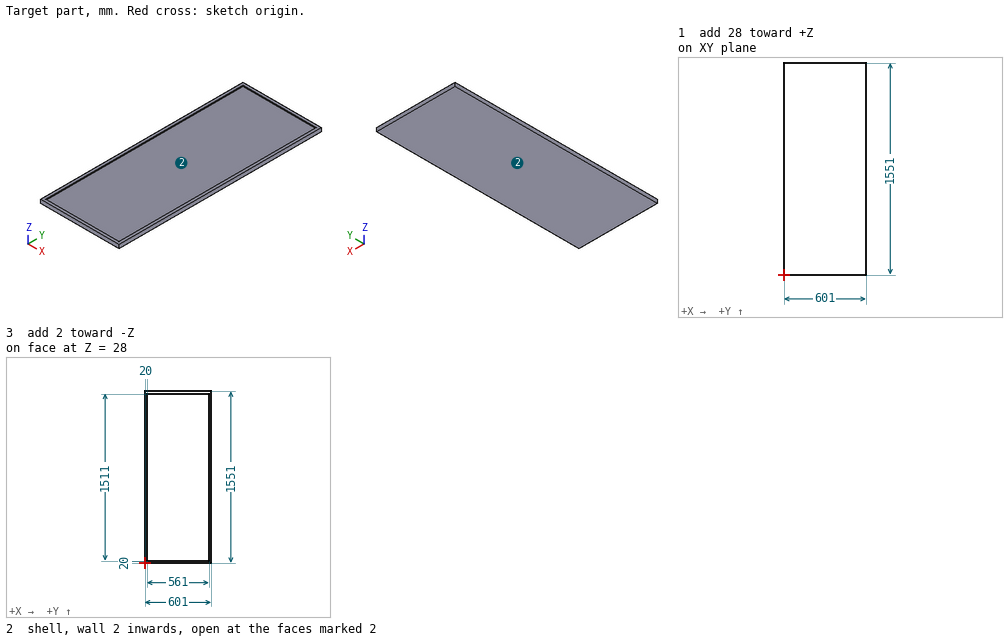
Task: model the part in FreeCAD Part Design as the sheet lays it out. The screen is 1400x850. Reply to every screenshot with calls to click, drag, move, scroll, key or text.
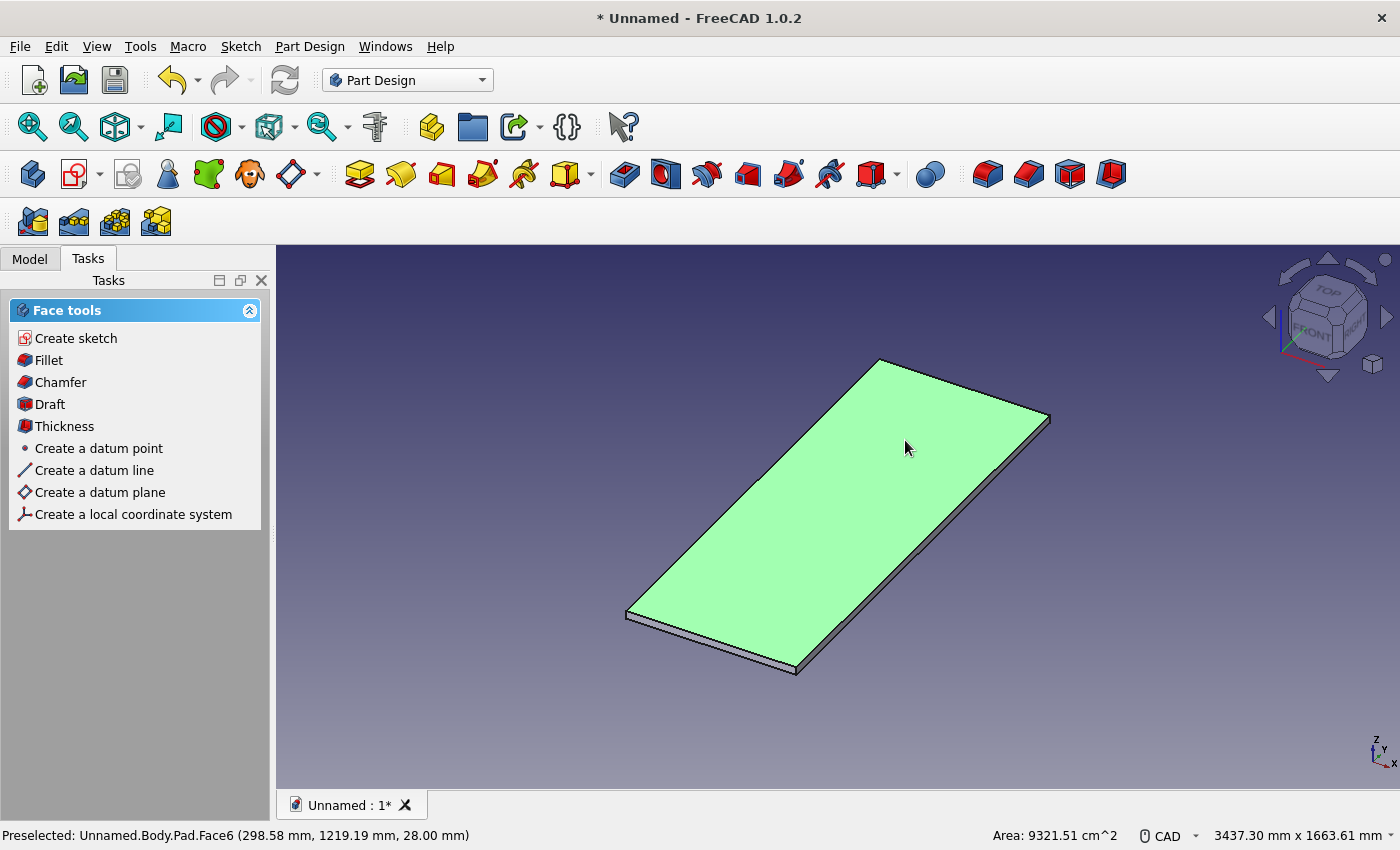
click(1111, 174)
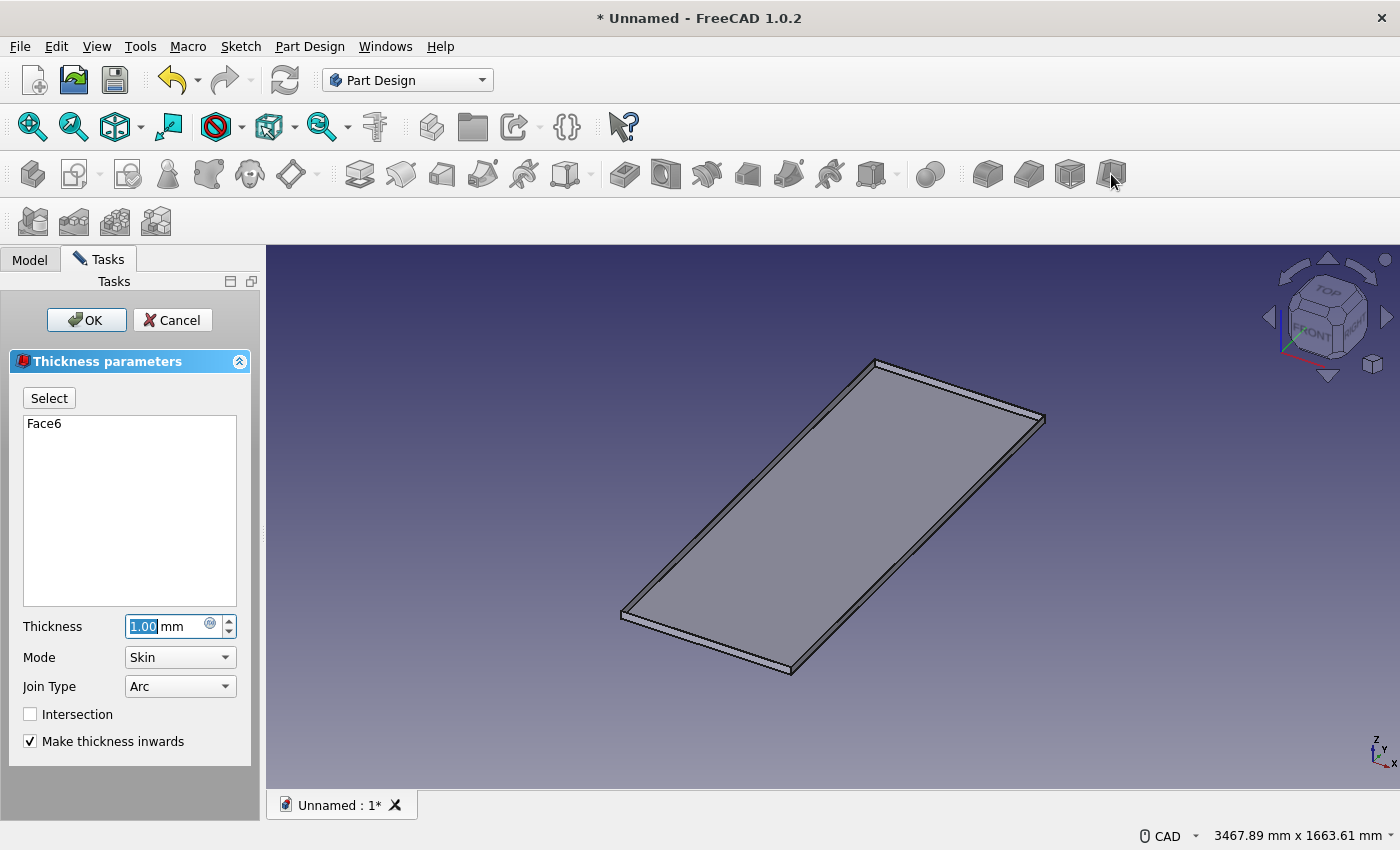
text(2)
key(Tab)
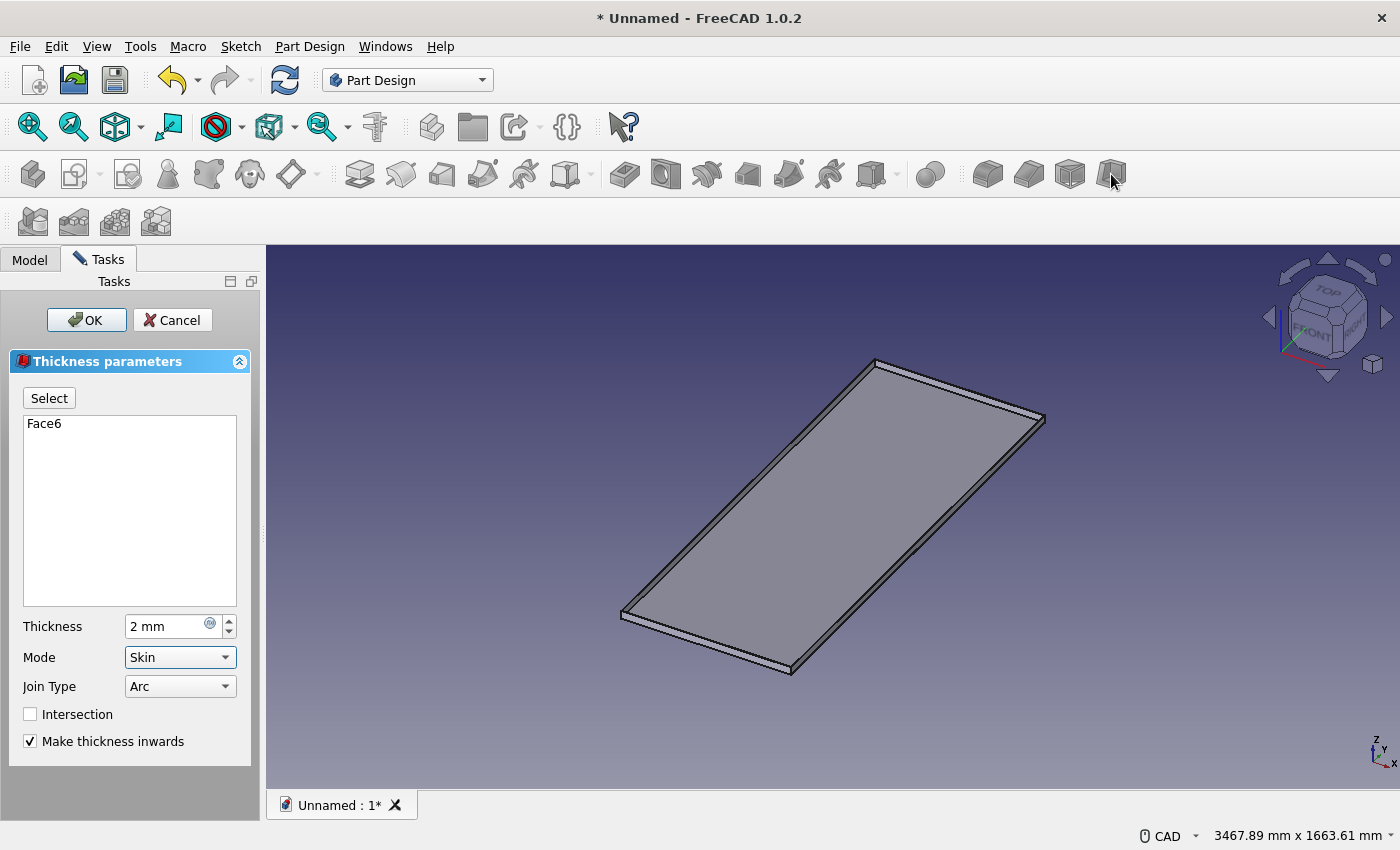
click(181, 686)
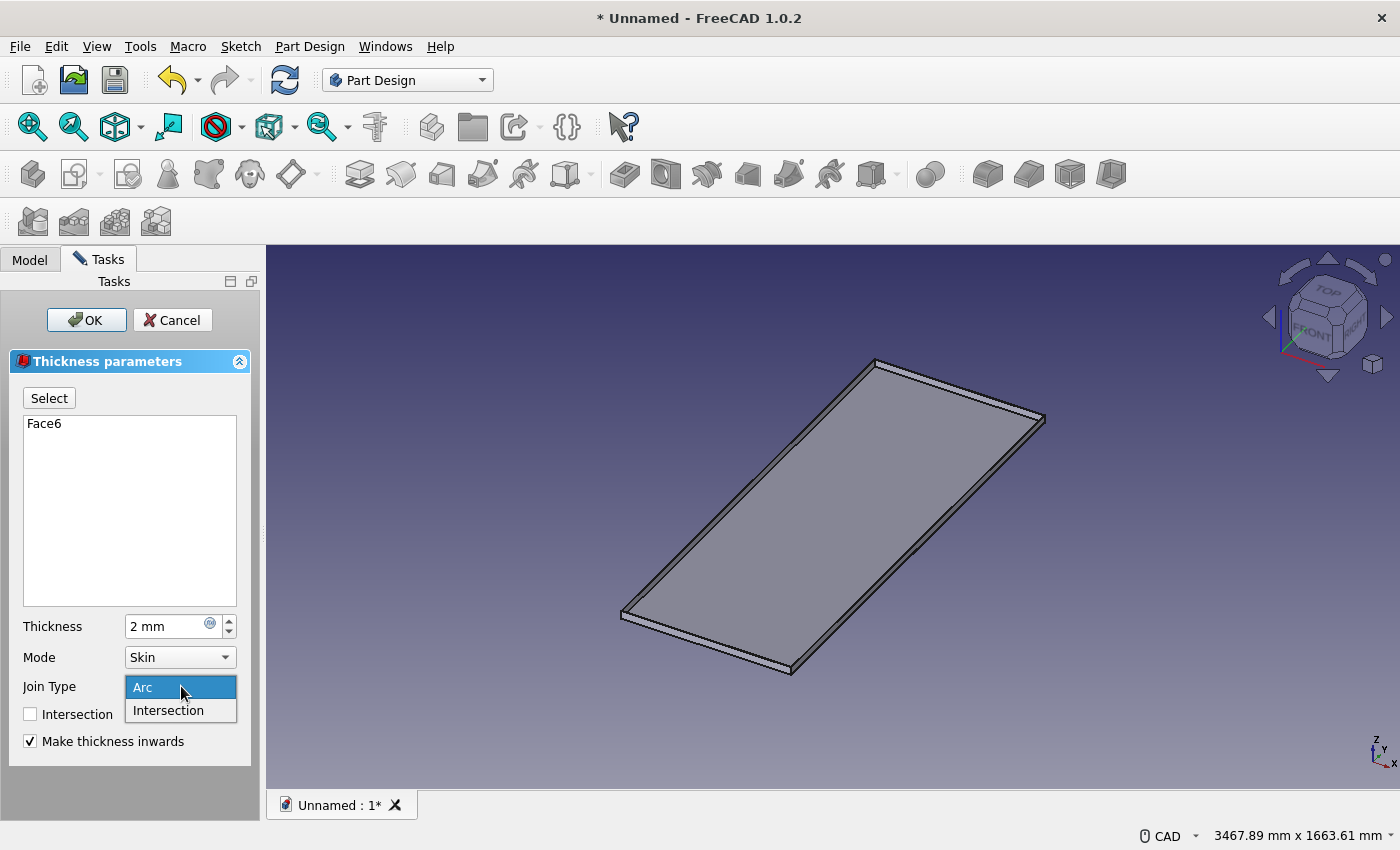
click(179, 710)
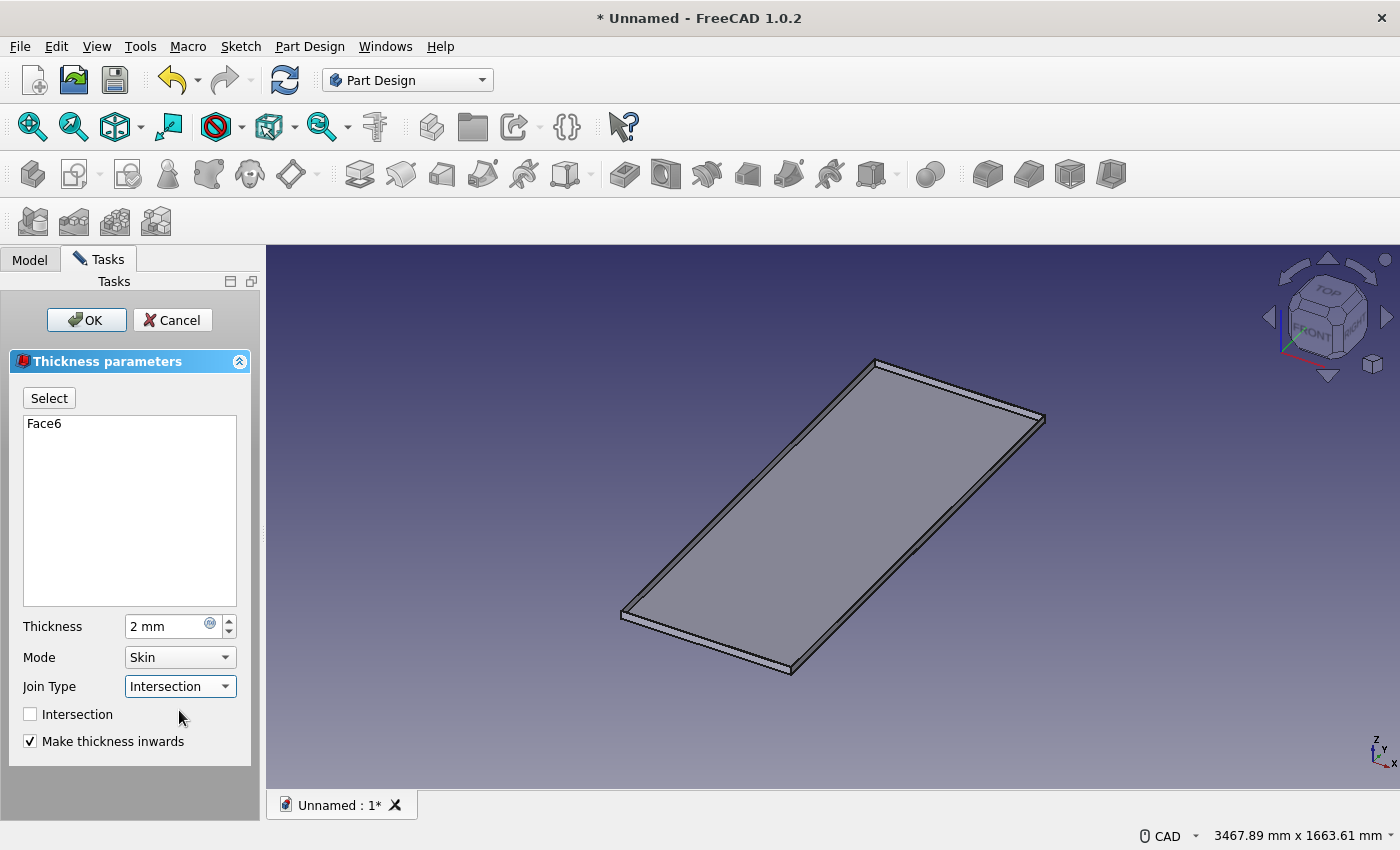
click(87, 320)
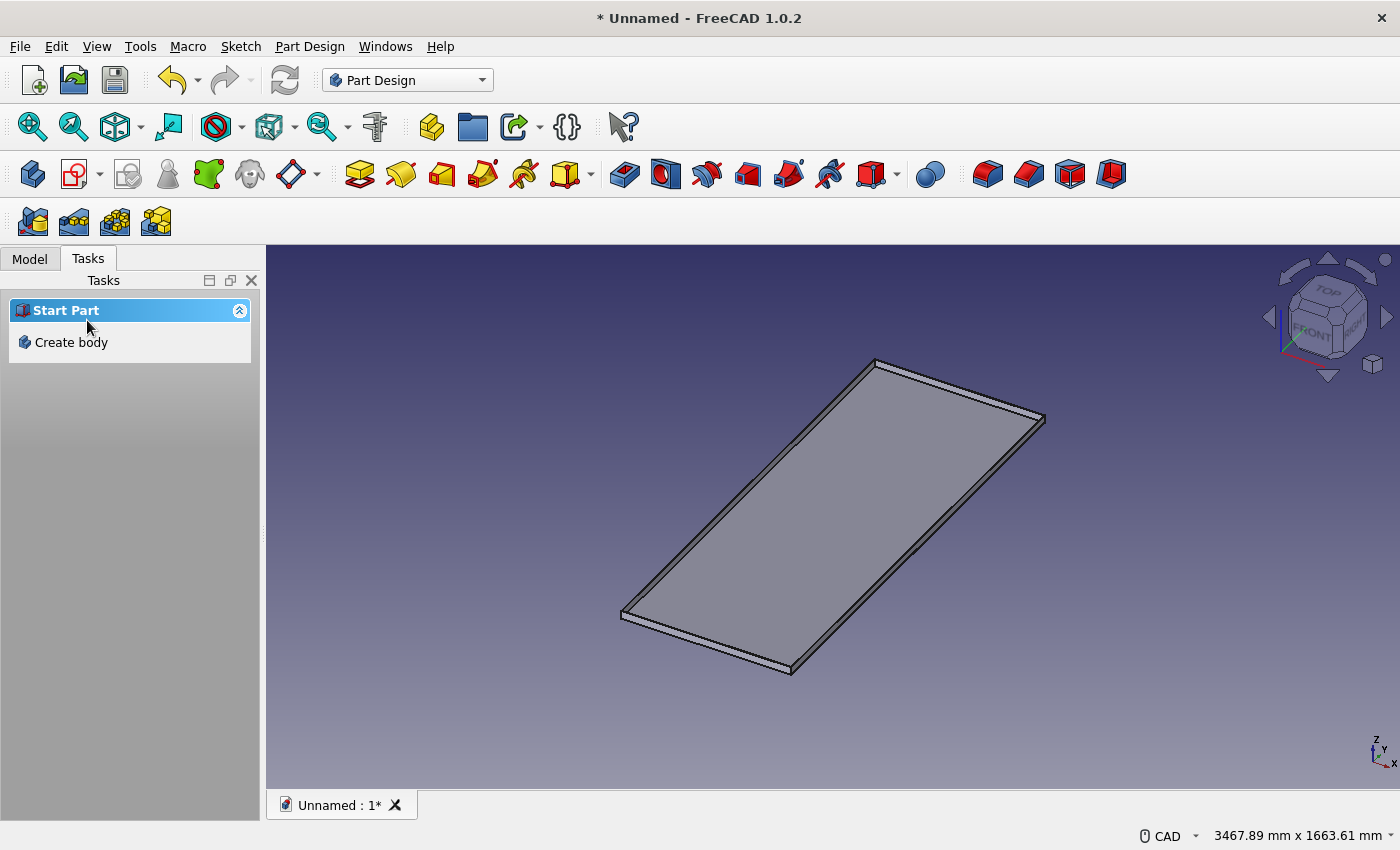
scroll(988, 396, up, 15)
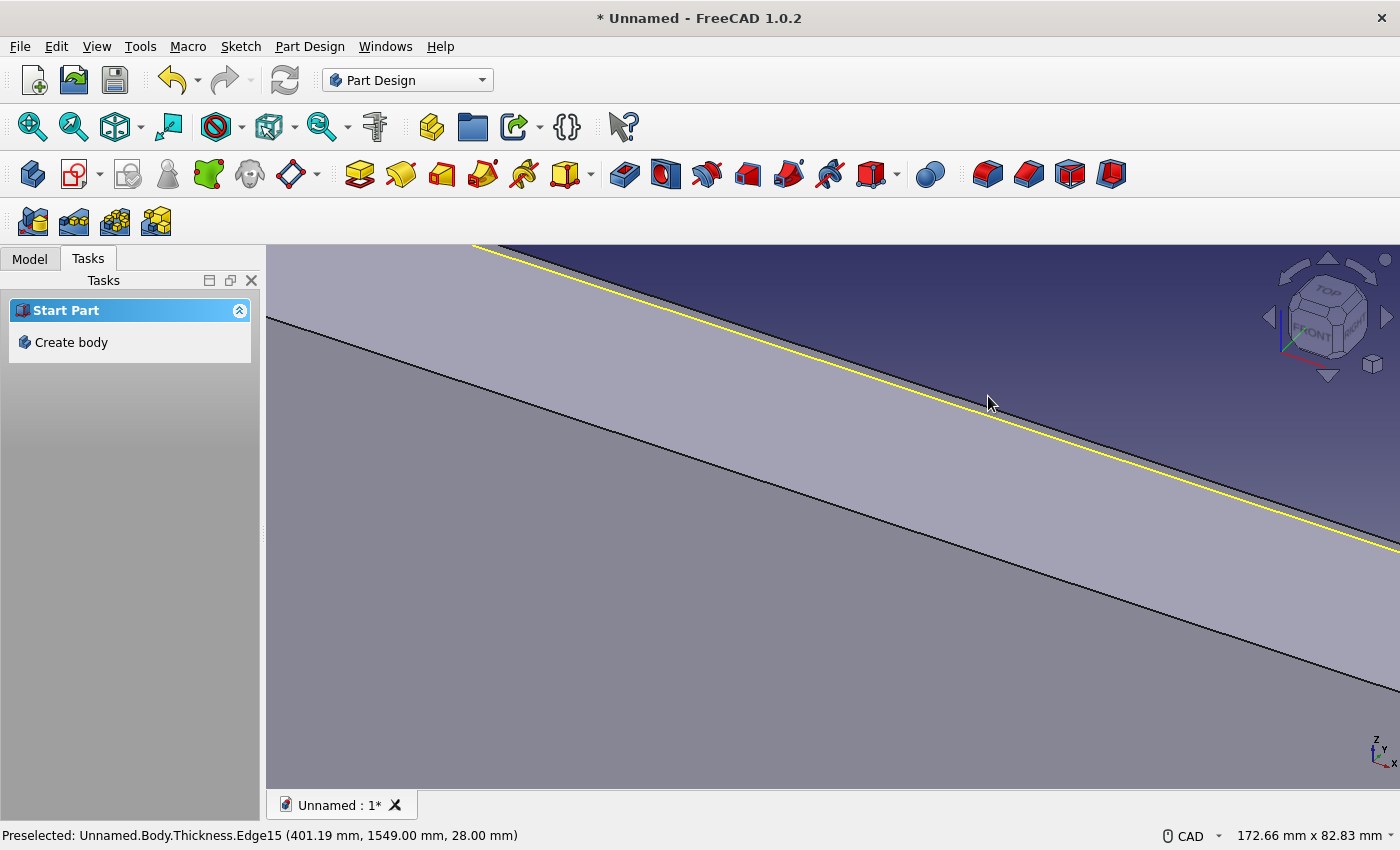
scroll(975, 408, up, 6)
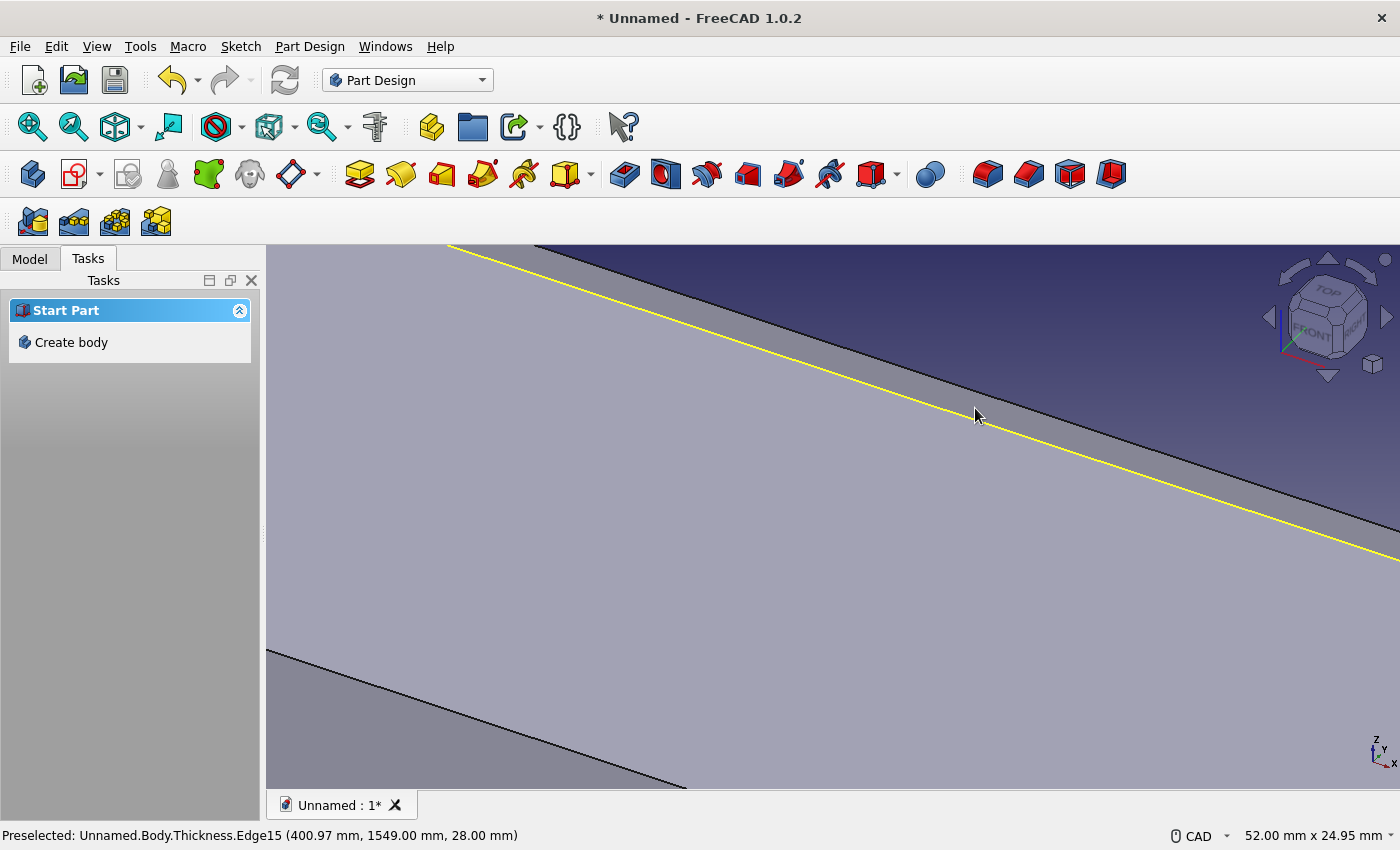
click(972, 408)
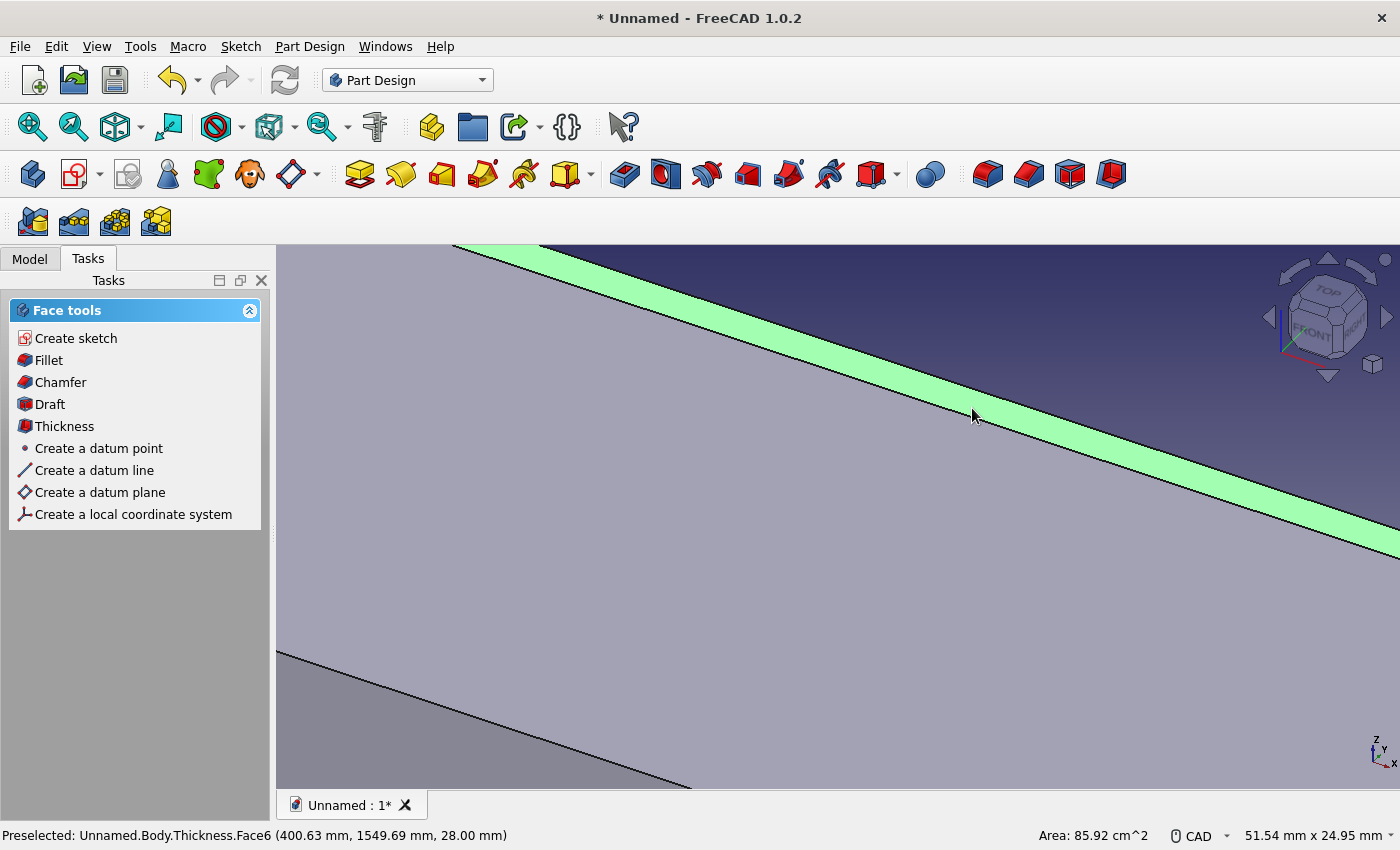
click(74, 174)